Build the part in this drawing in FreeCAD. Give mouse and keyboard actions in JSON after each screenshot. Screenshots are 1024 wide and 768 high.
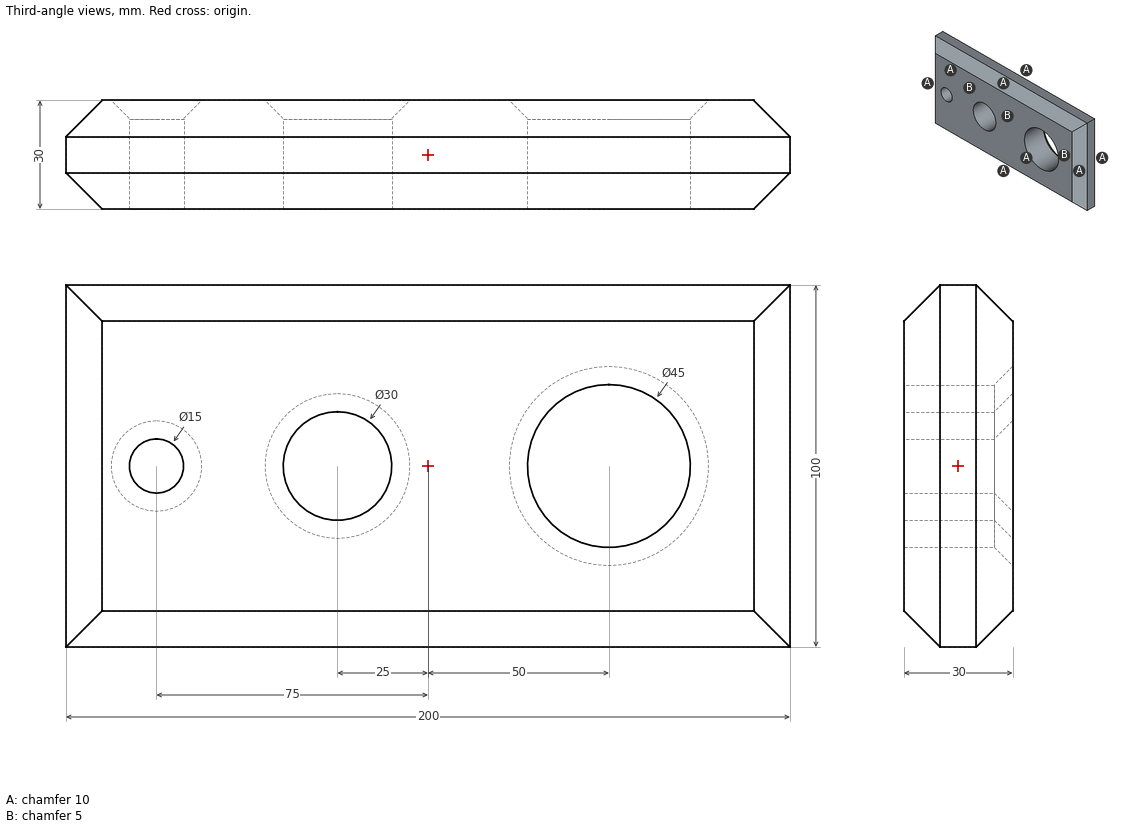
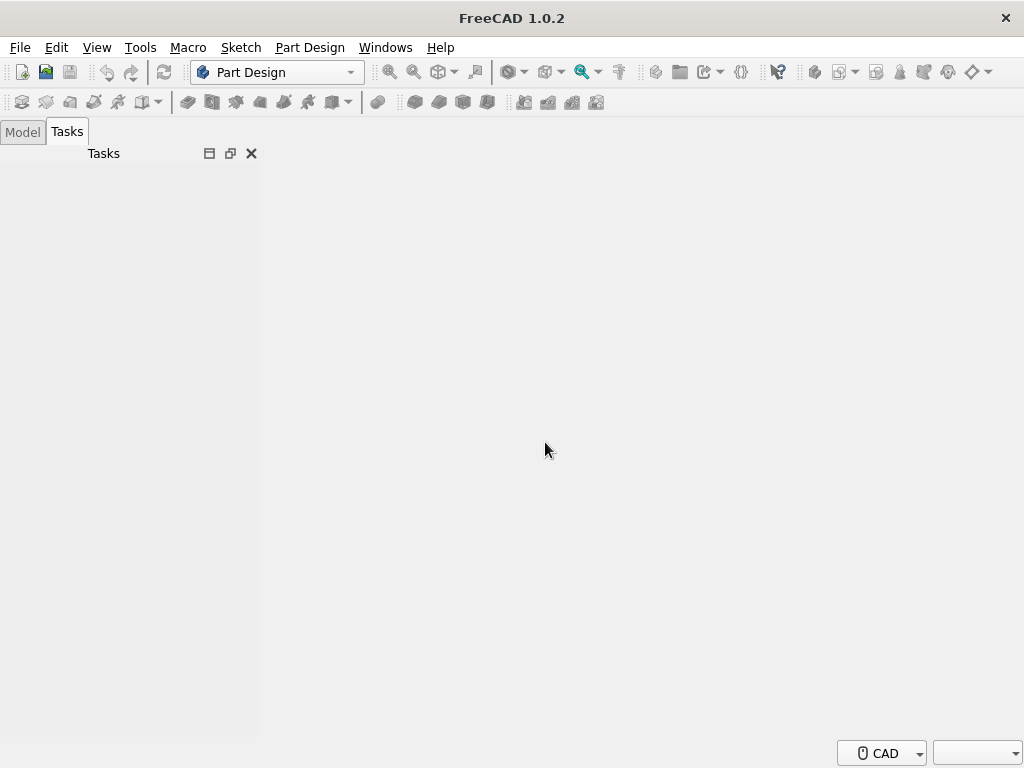
{"action": "key", "text": "ctrl+n"}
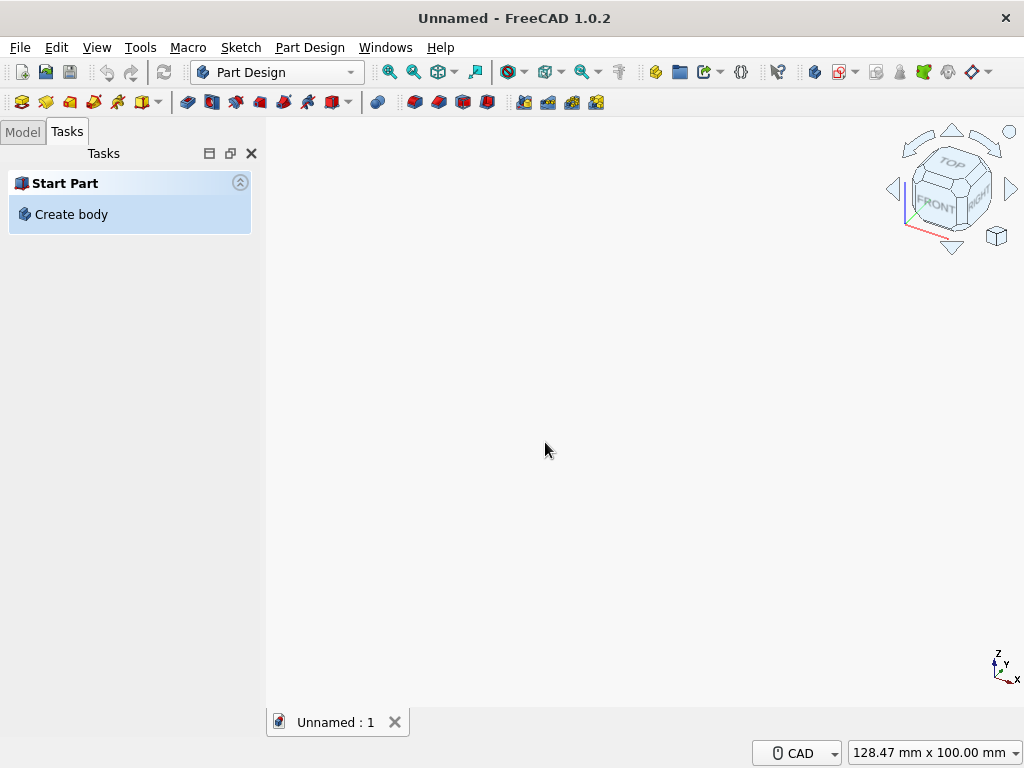
{"action": "left_click", "coordinate": [840, 72]}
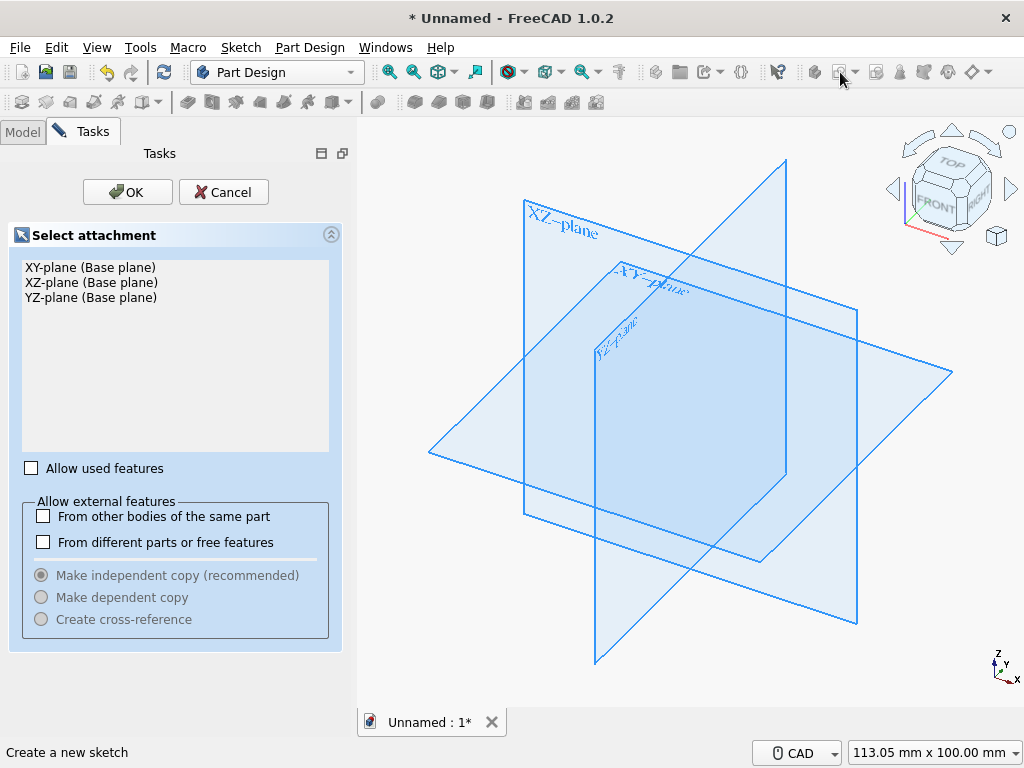
{"action": "left_click", "coordinate": [82, 282]}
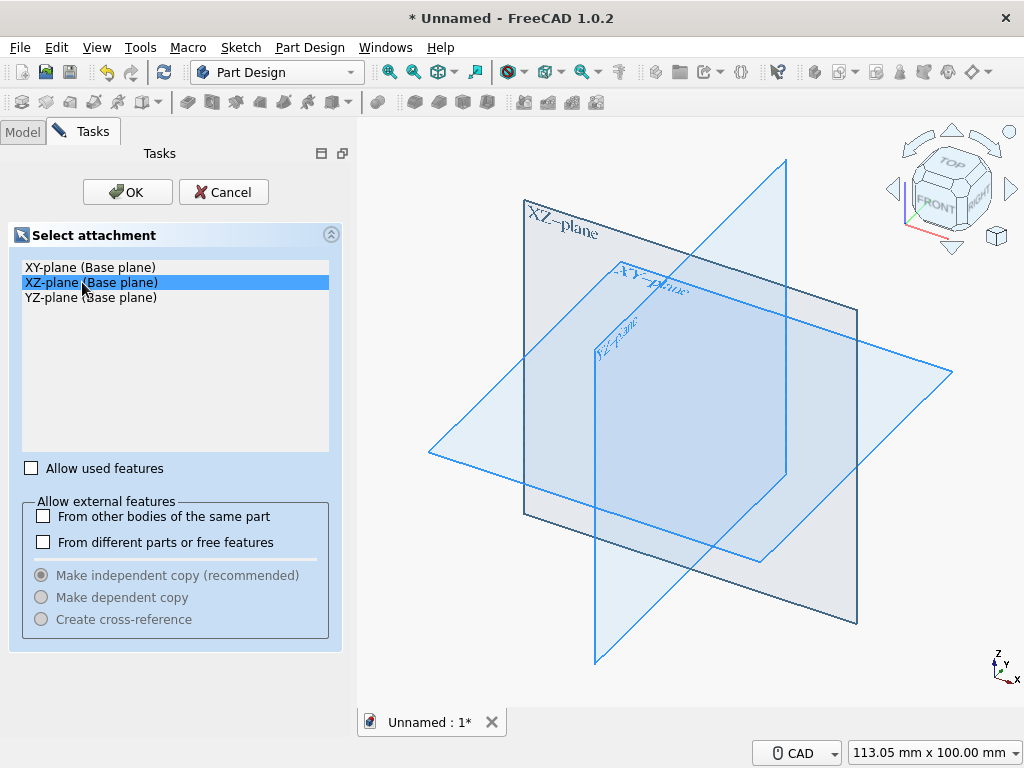
{"action": "left_click", "coordinate": [128, 192]}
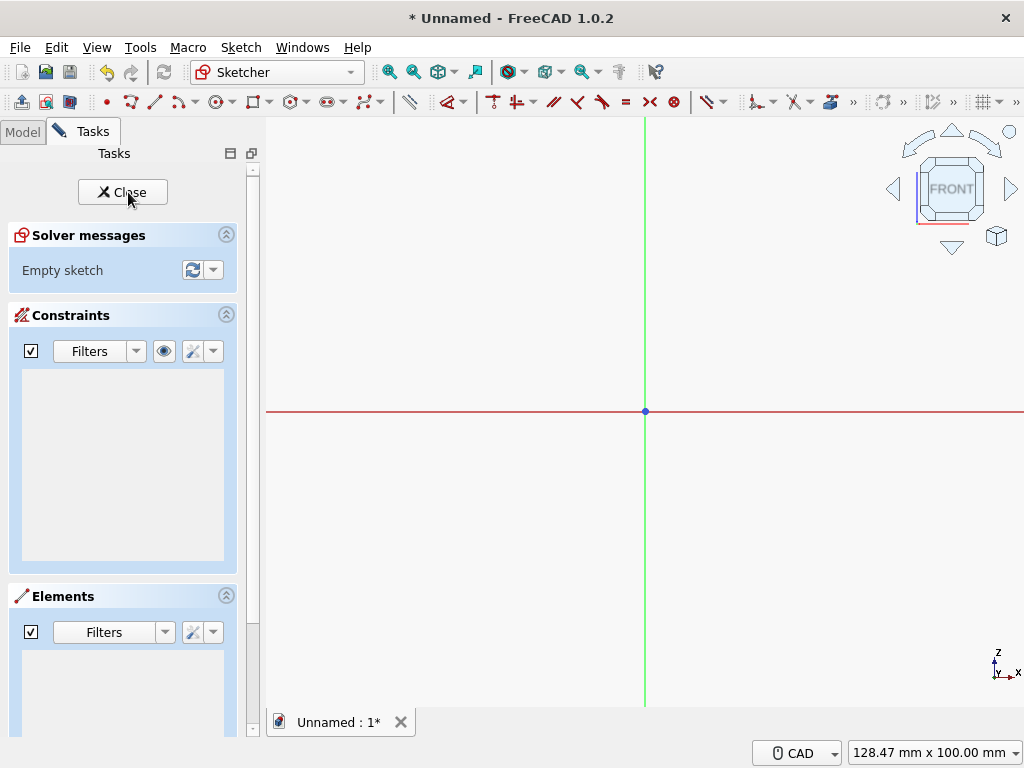
{"action": "scroll", "coordinate": [537, 412], "scroll_direction": "down", "scroll_amount": 5}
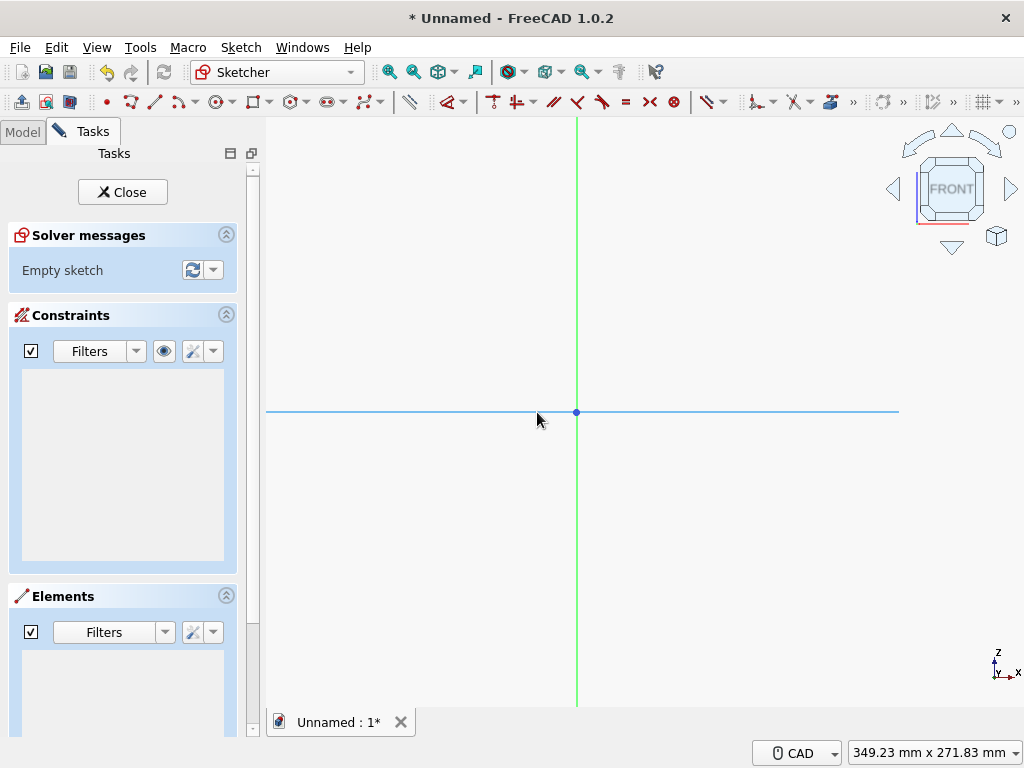
{"action": "left_click", "coordinate": [272, 102]}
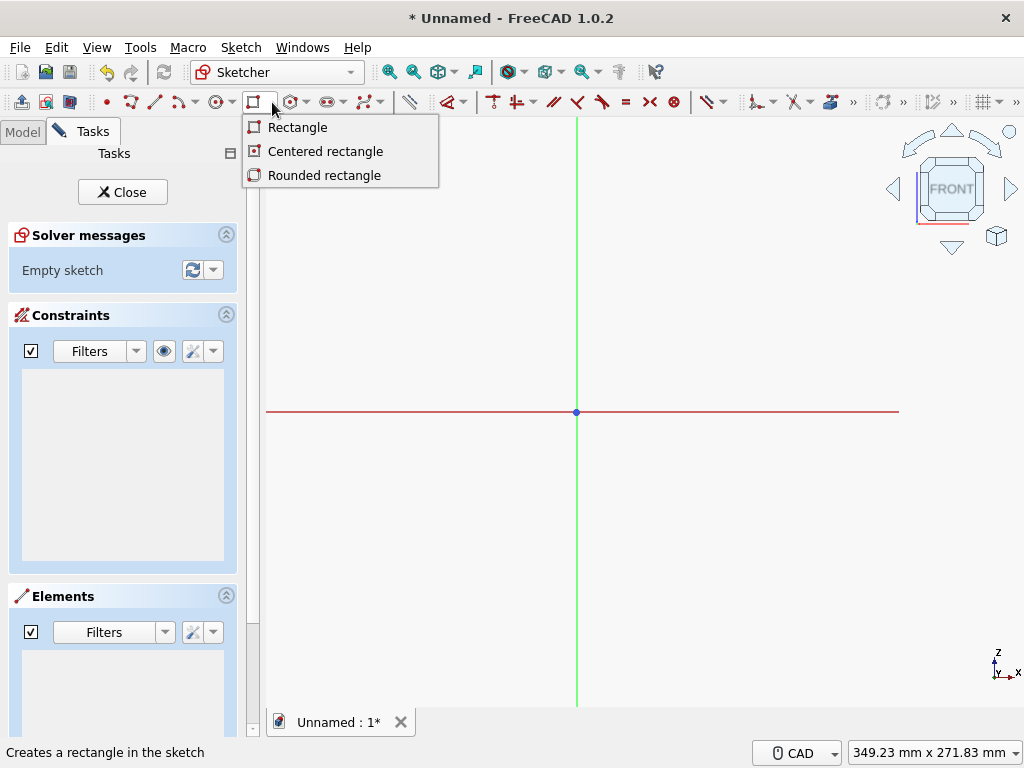
{"action": "left_click", "coordinate": [340, 151]}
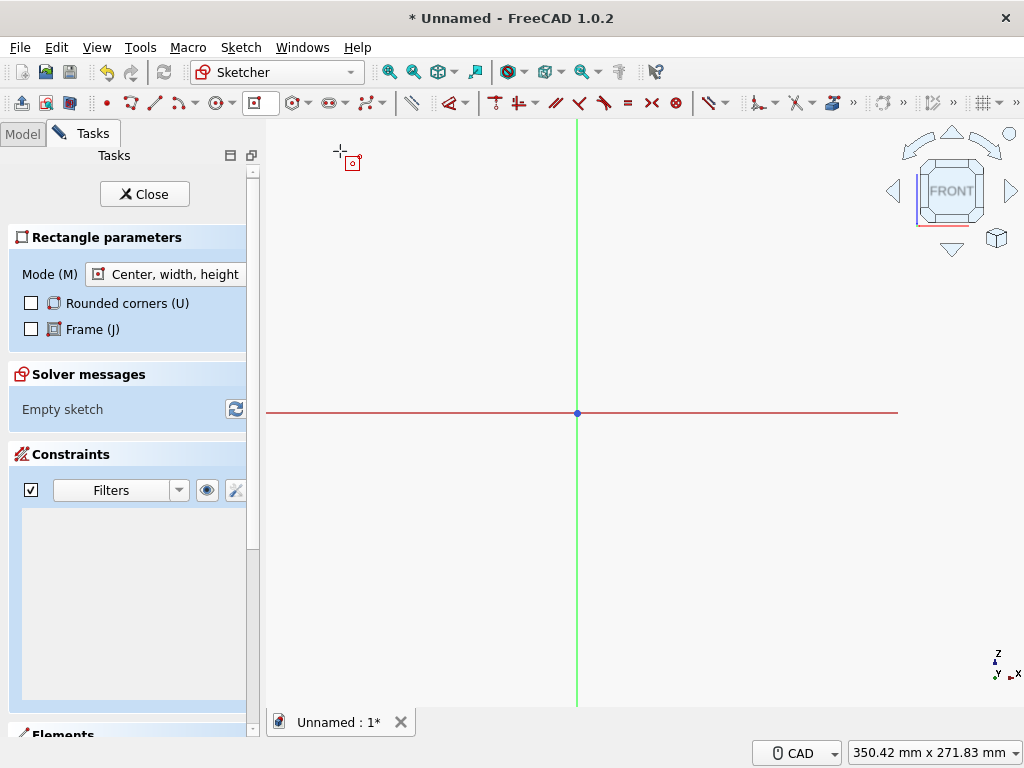
{"action": "left_click", "coordinate": [577, 413]}
{"action": "left_click", "coordinate": [794, 305]}
{"action": "key", "text": "Escape"}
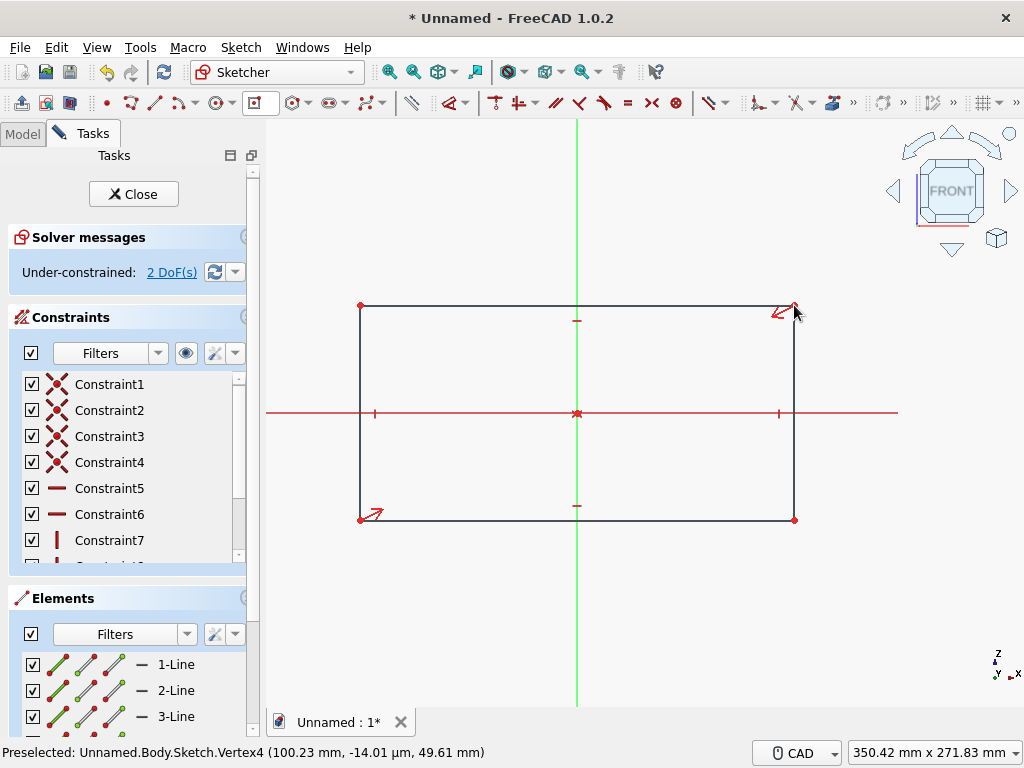
{"action": "left_click", "coordinate": [450, 104]}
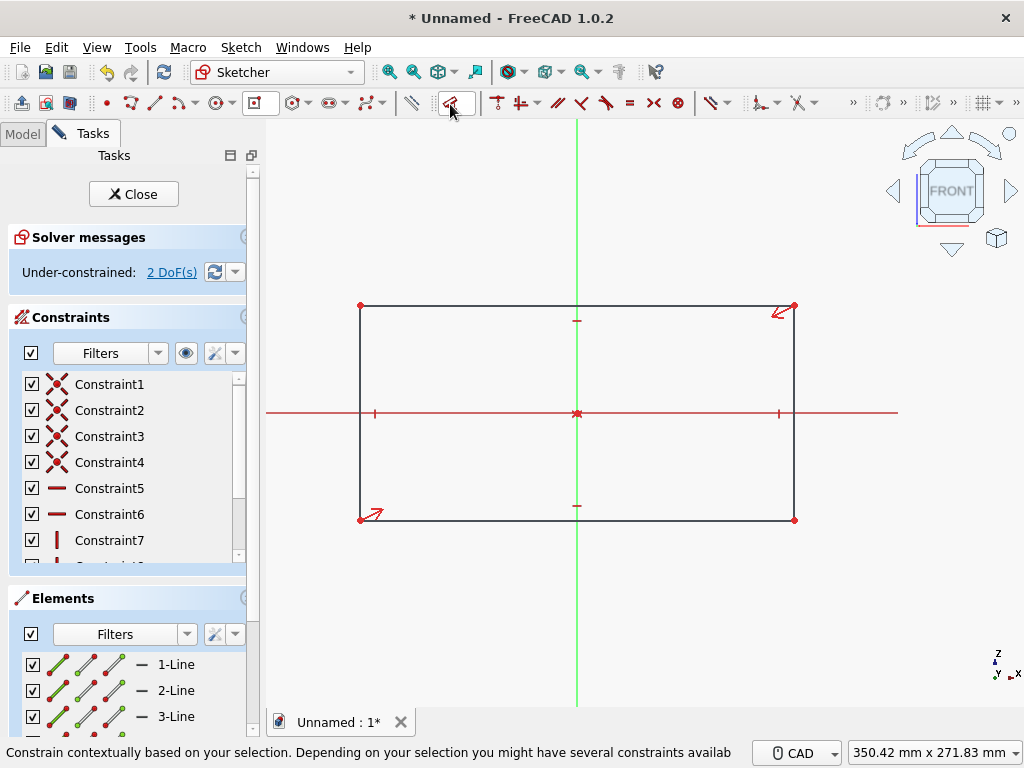
{"action": "left_click", "coordinate": [490, 521]}
{"action": "left_click", "coordinate": [477, 555]}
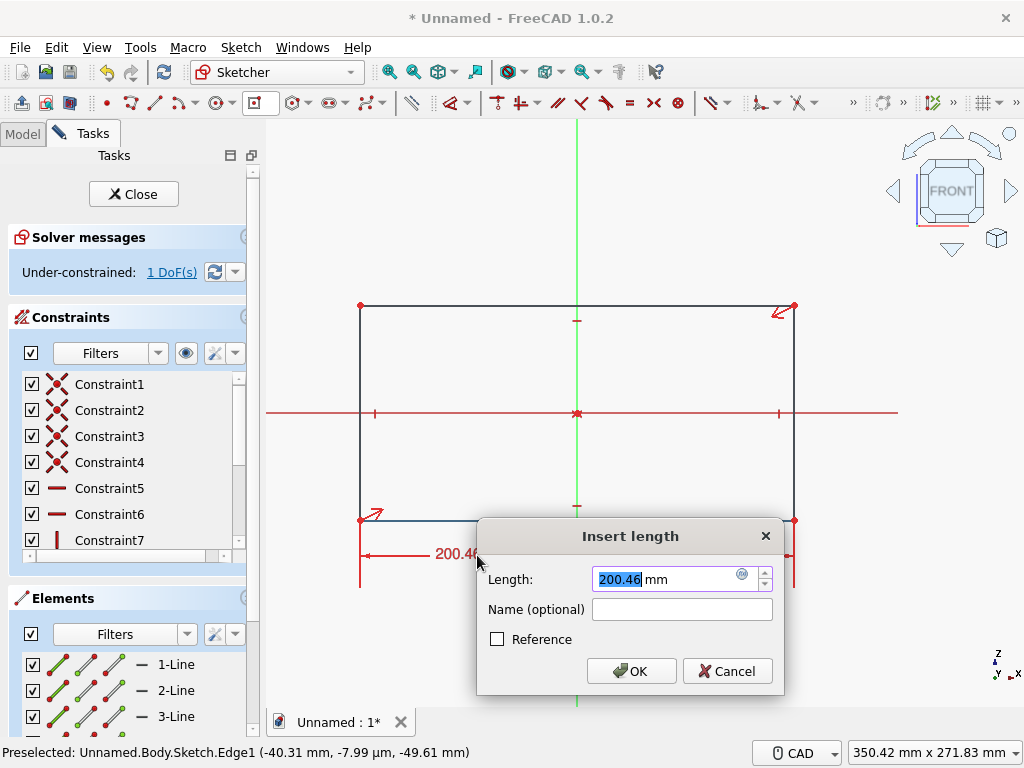
{"action": "type", "text": "200"}
{"action": "key", "text": "Return"}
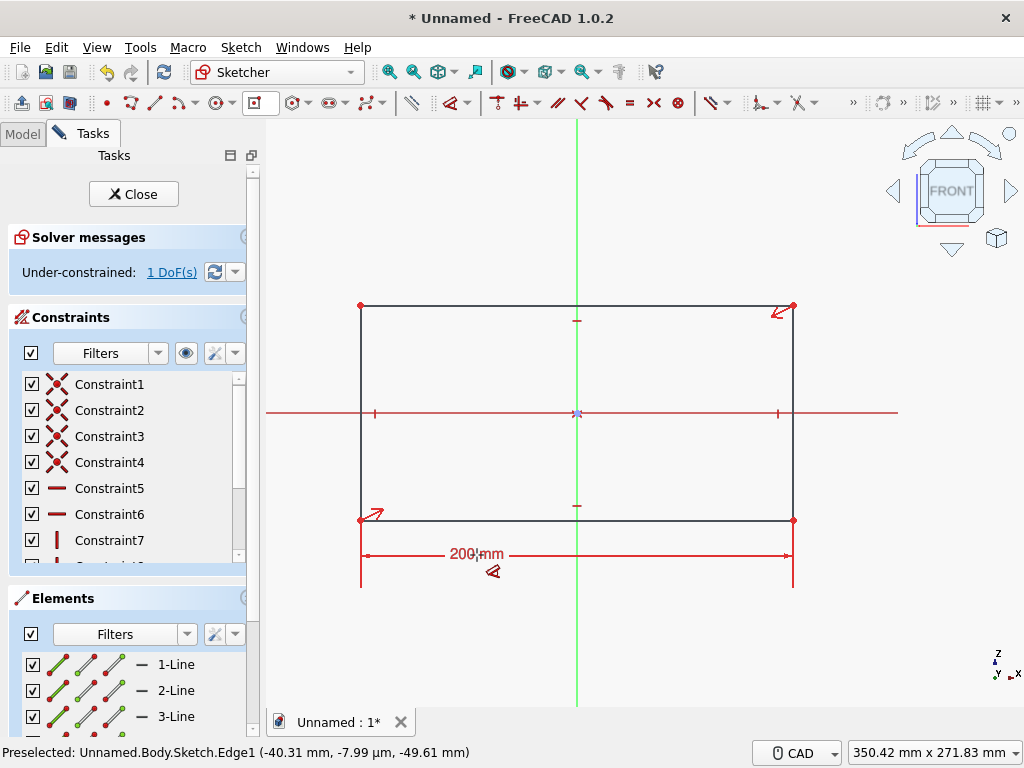
{"action": "left_click", "coordinate": [794, 456]}
{"action": "left_click", "coordinate": [828, 364]}